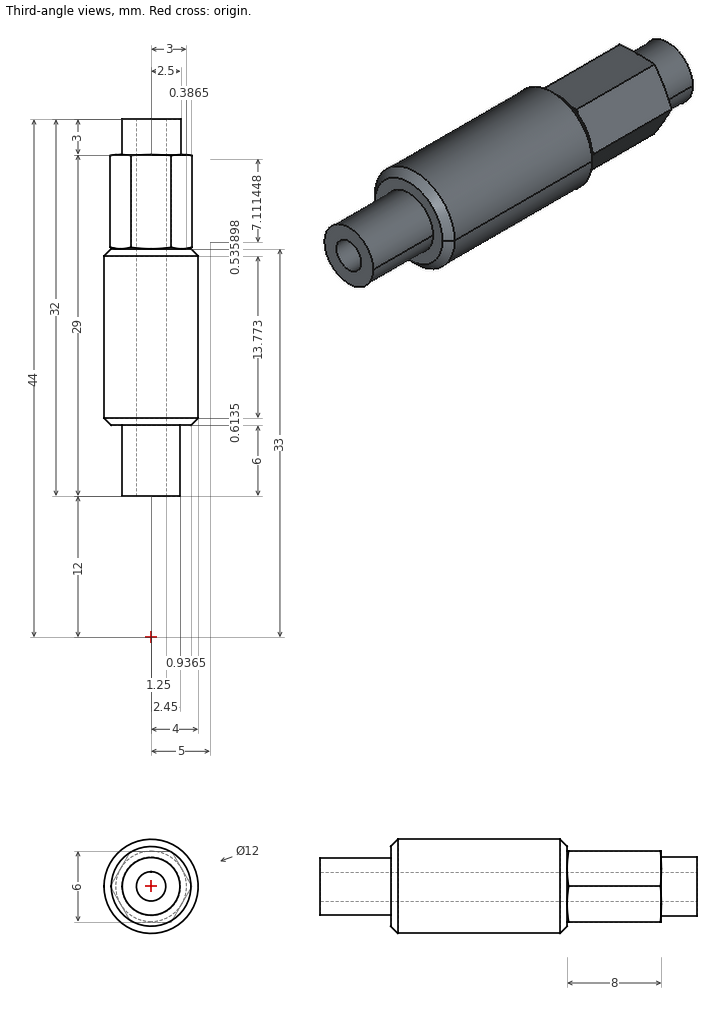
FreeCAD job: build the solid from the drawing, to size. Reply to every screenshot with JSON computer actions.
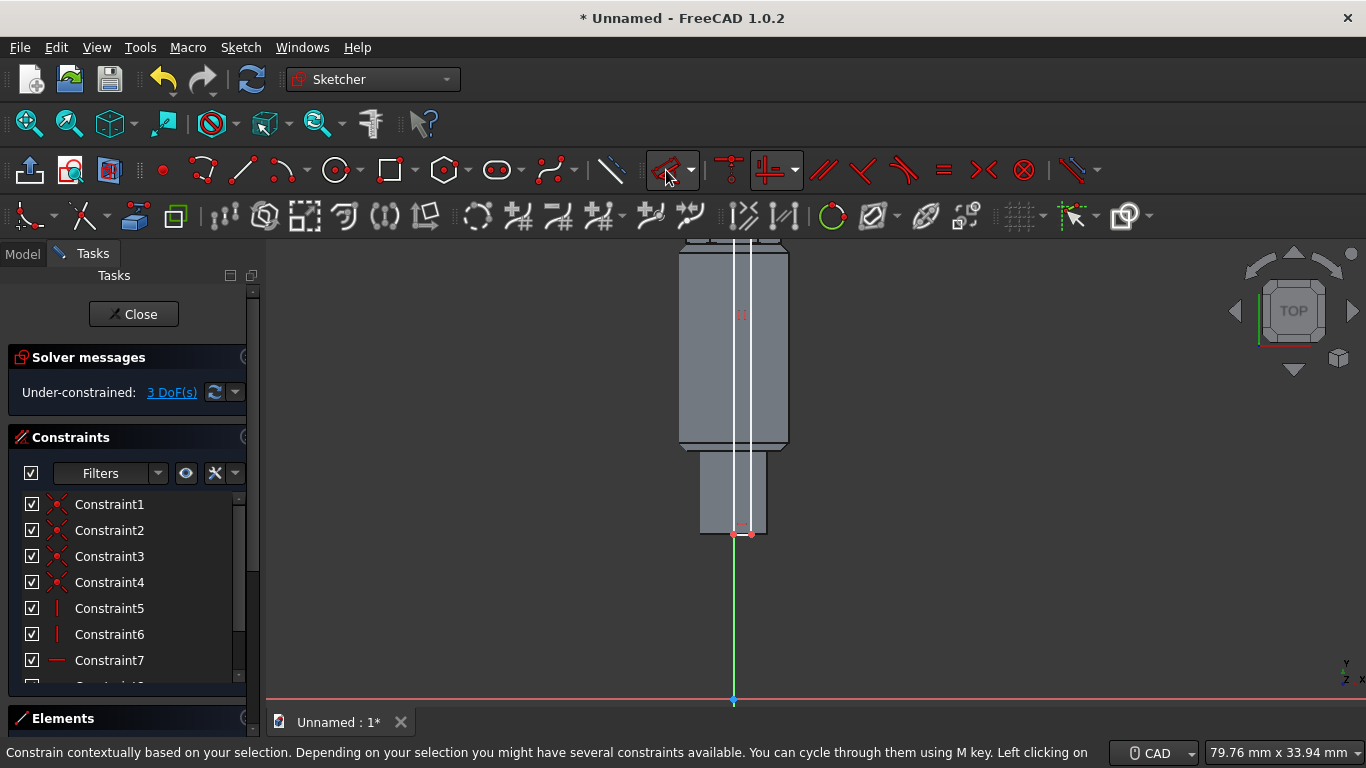
{"action": "left_click", "coordinate": [734, 403]}
{"action": "left_click", "coordinate": [700, 401]}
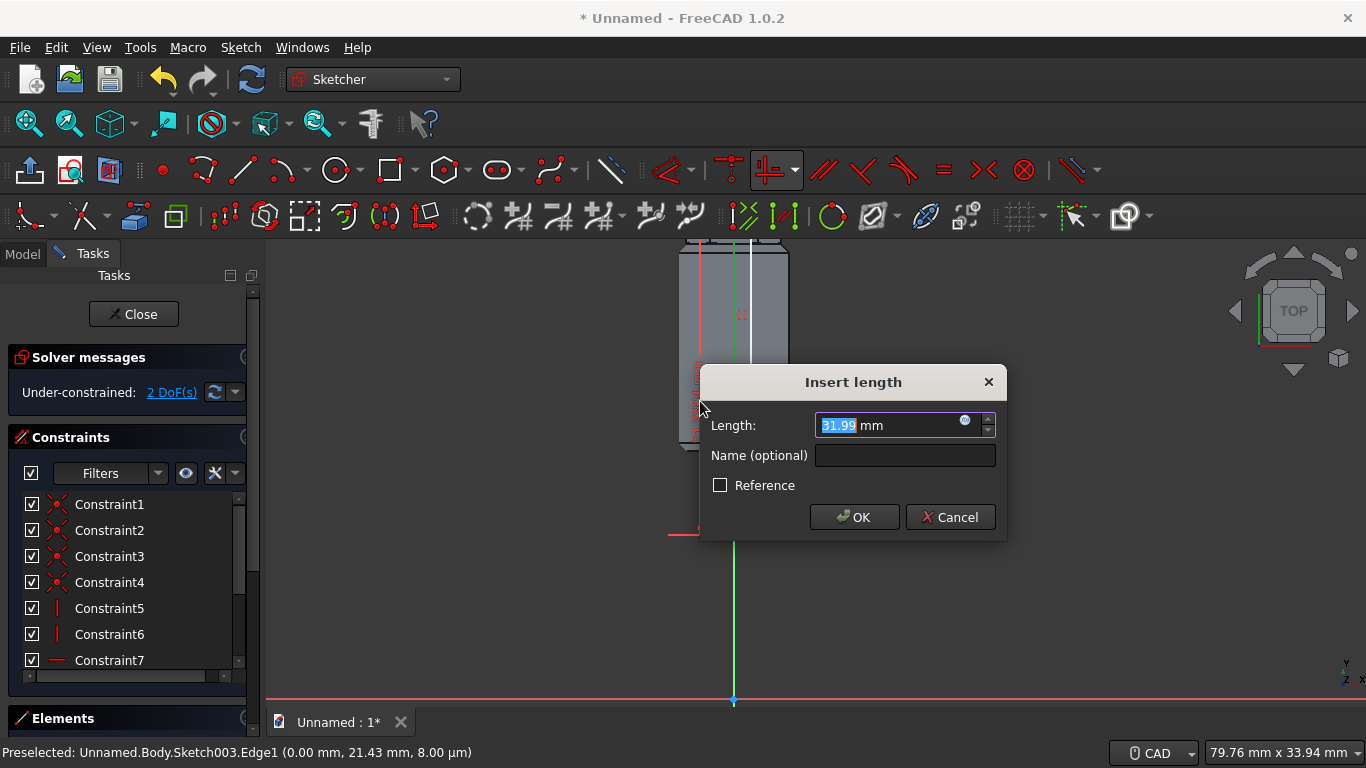
{"action": "type", "text": "32"}
{"action": "key", "text": "Return"}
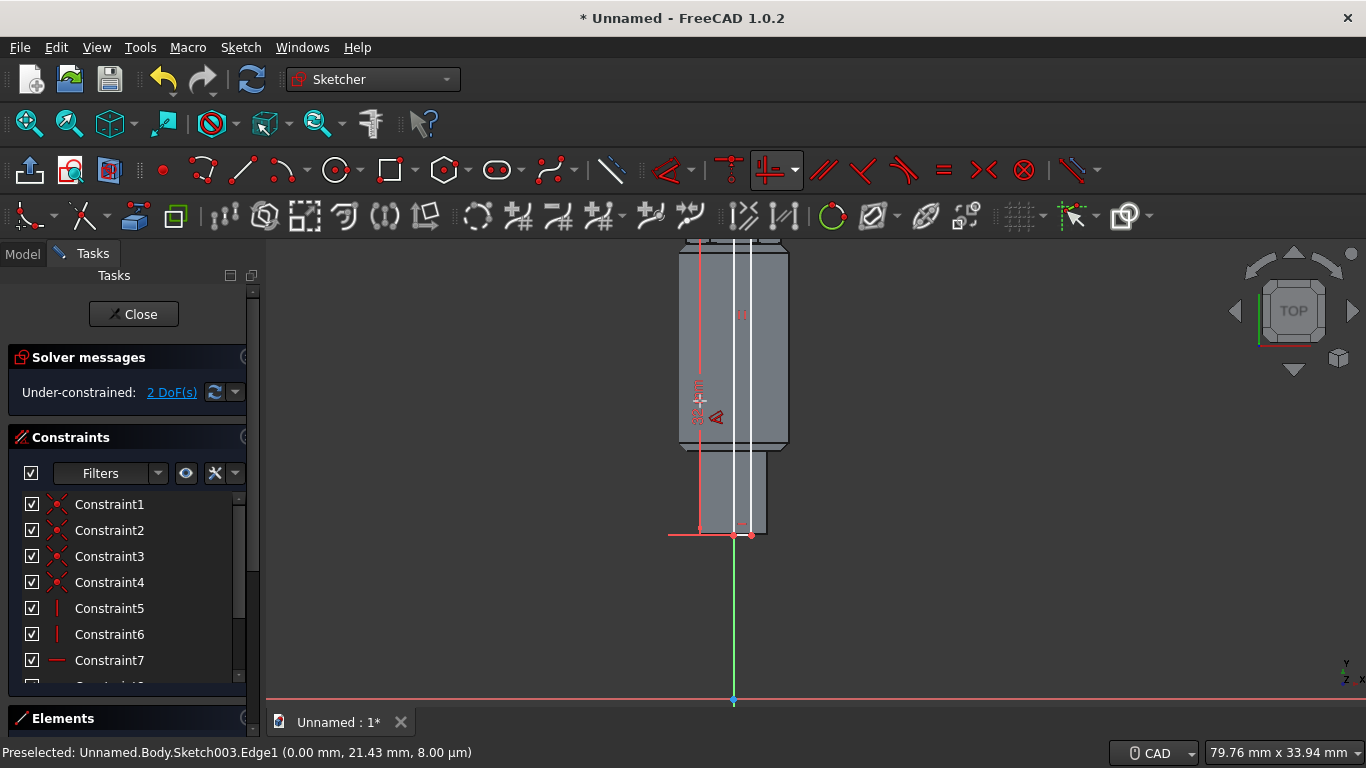
{"action": "scroll", "coordinate": [752, 536], "scroll_direction": "down", "scroll_amount": 4}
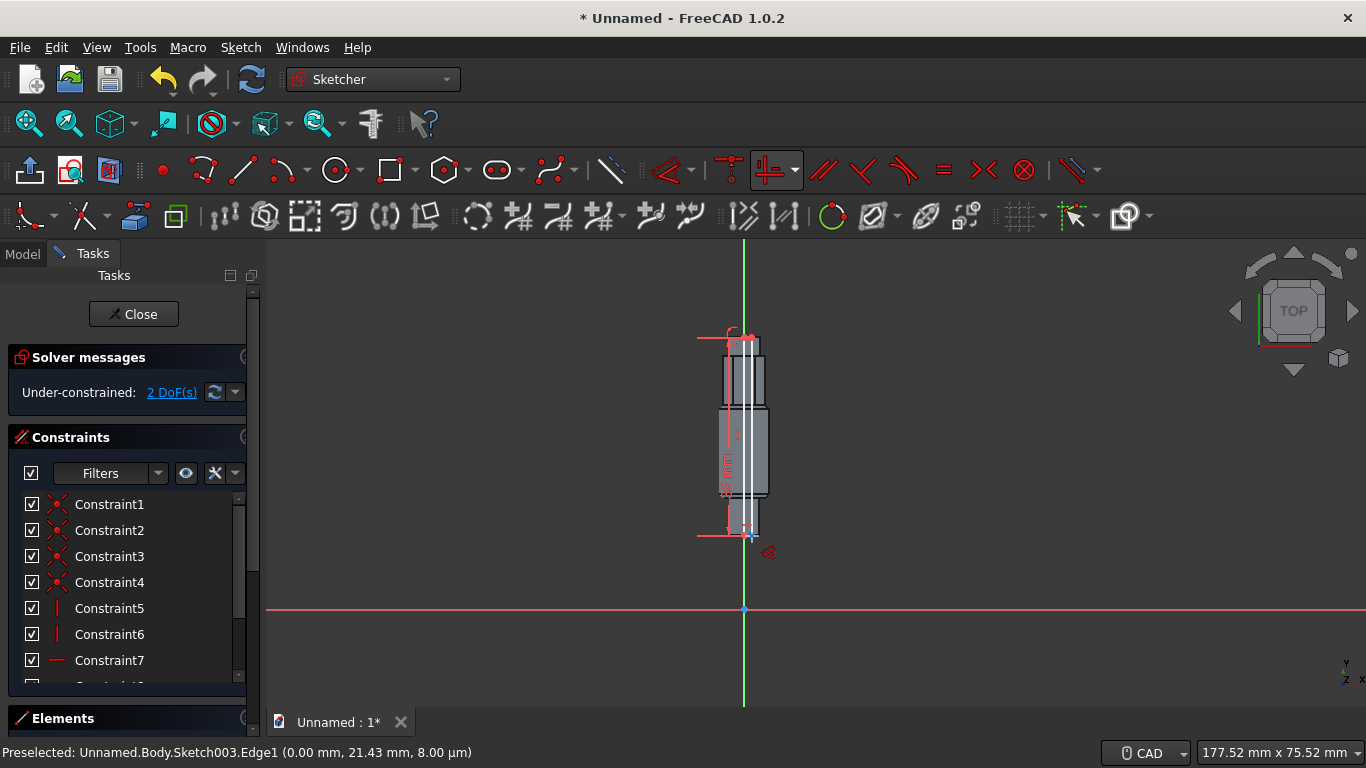
{"action": "scroll", "coordinate": [744, 338], "scroll_direction": "up", "scroll_amount": 3}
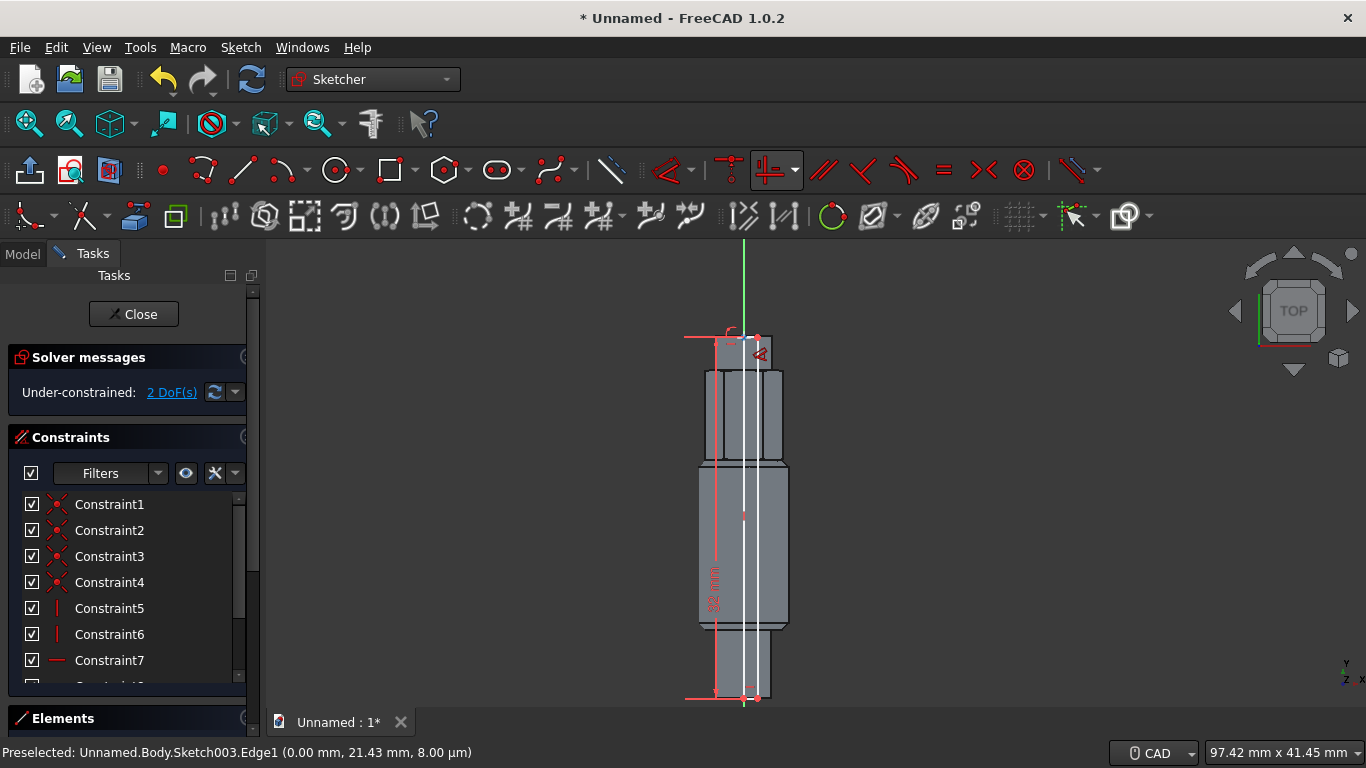
{"action": "left_click", "coordinate": [744, 337]}
{"action": "left_click", "coordinate": [710, 508]}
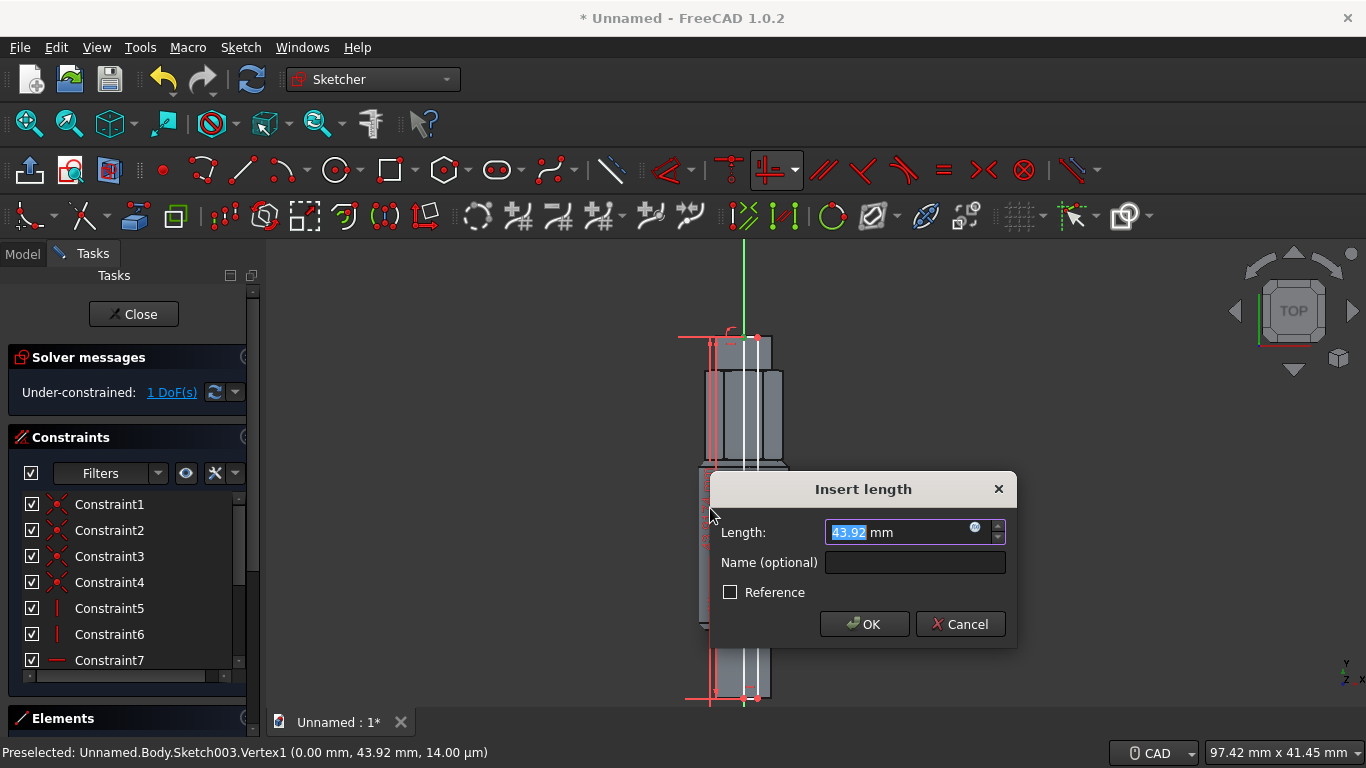
{"action": "type", "text": "44"}
{"action": "key", "text": "Return"}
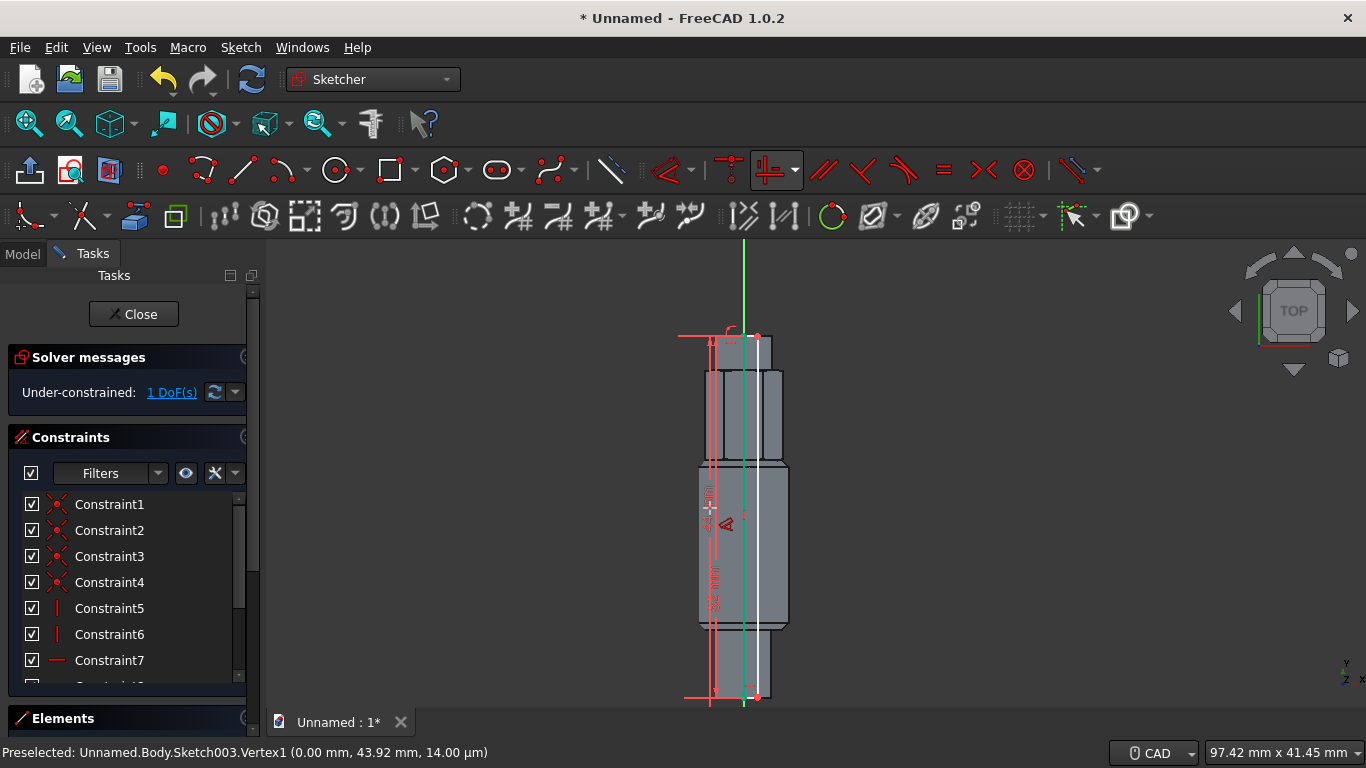
{"action": "scroll", "coordinate": [744, 337], "scroll_direction": "down", "scroll_amount": 3}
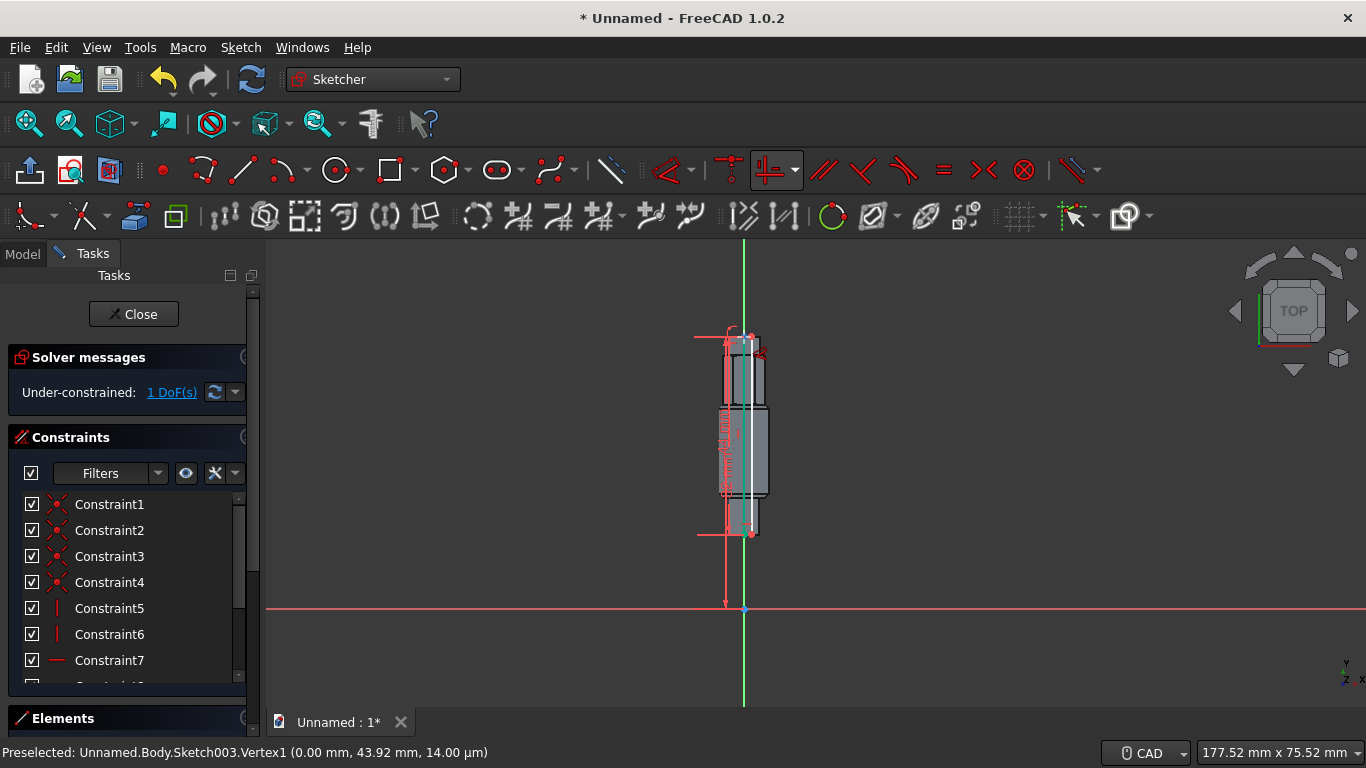
{"action": "scroll", "coordinate": [748, 535], "scroll_direction": "up", "scroll_amount": 9}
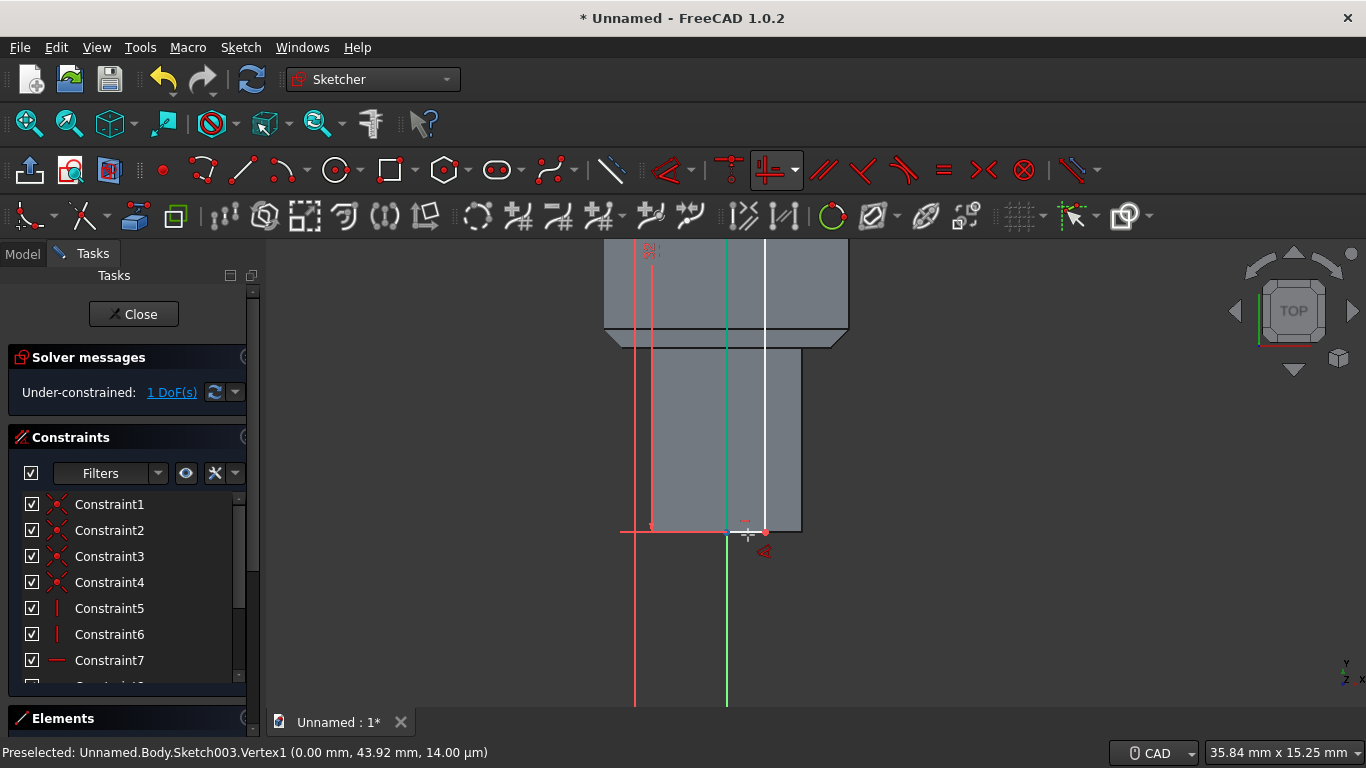
{"action": "left_click", "coordinate": [745, 532]}
{"action": "left_click", "coordinate": [745, 566]}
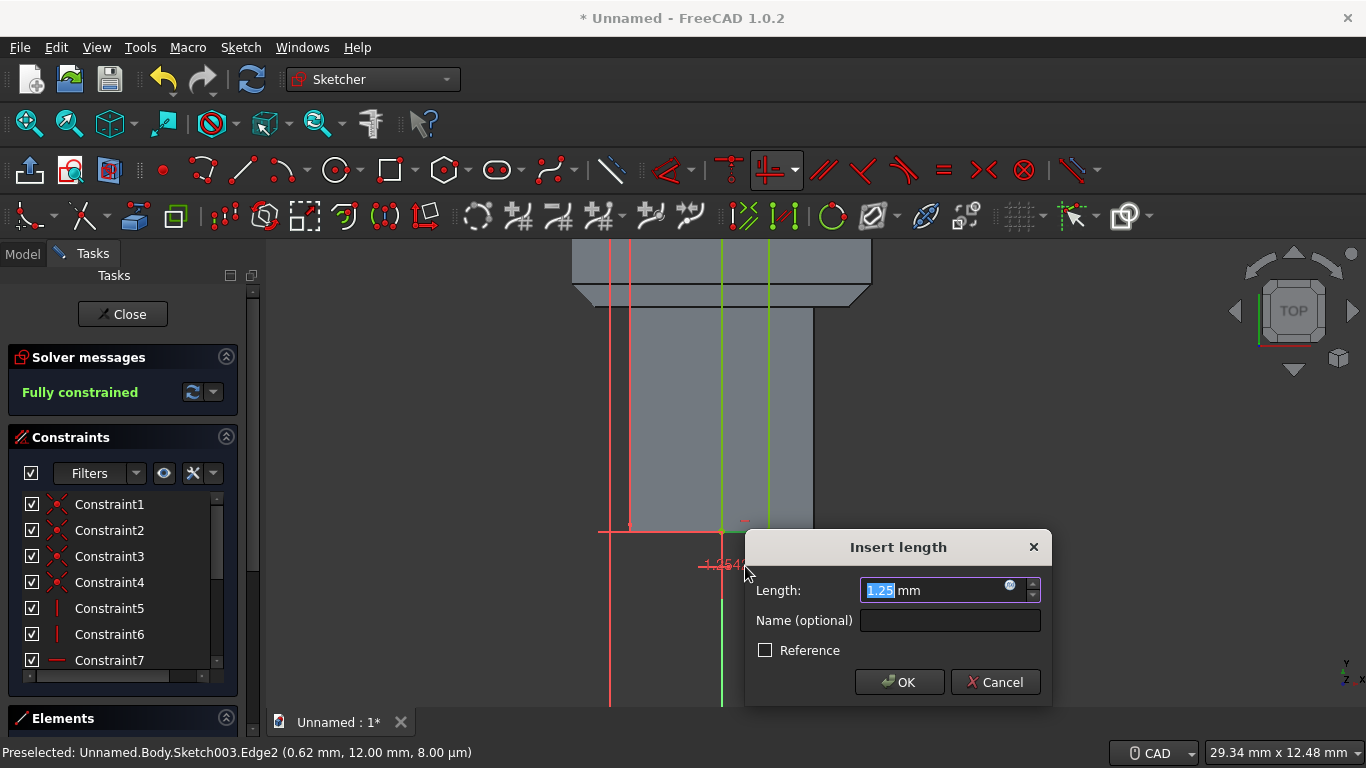
{"action": "type", "text": "1.25"}
{"action": "key", "text": "Return"}
{"action": "key", "text": "Escape"}